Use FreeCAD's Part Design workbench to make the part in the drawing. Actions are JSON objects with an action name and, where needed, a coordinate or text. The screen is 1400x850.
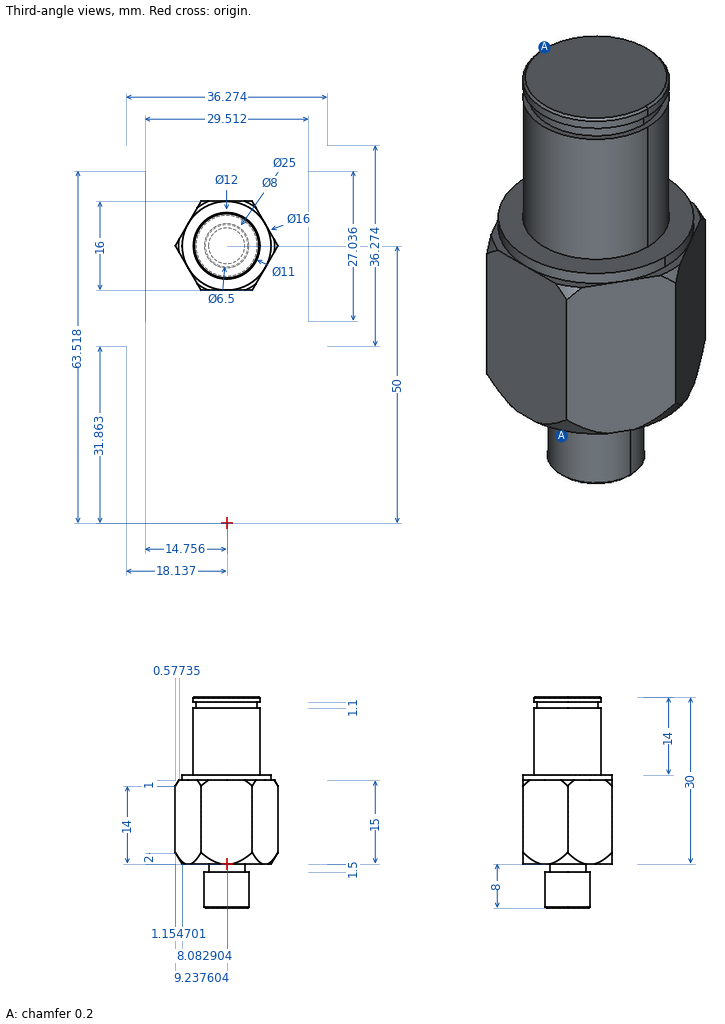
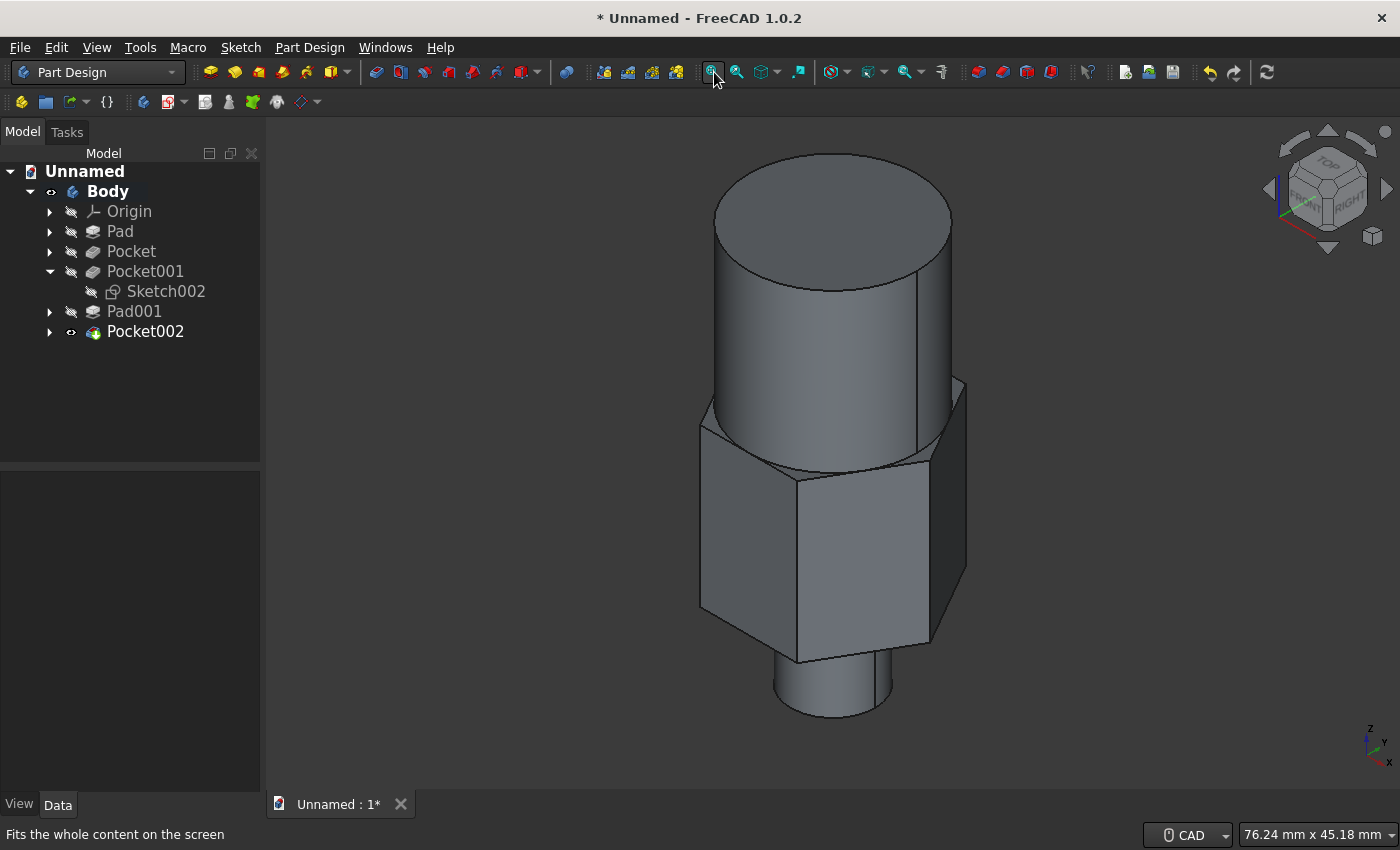
{"action": "left_click", "coordinate": [833, 221]}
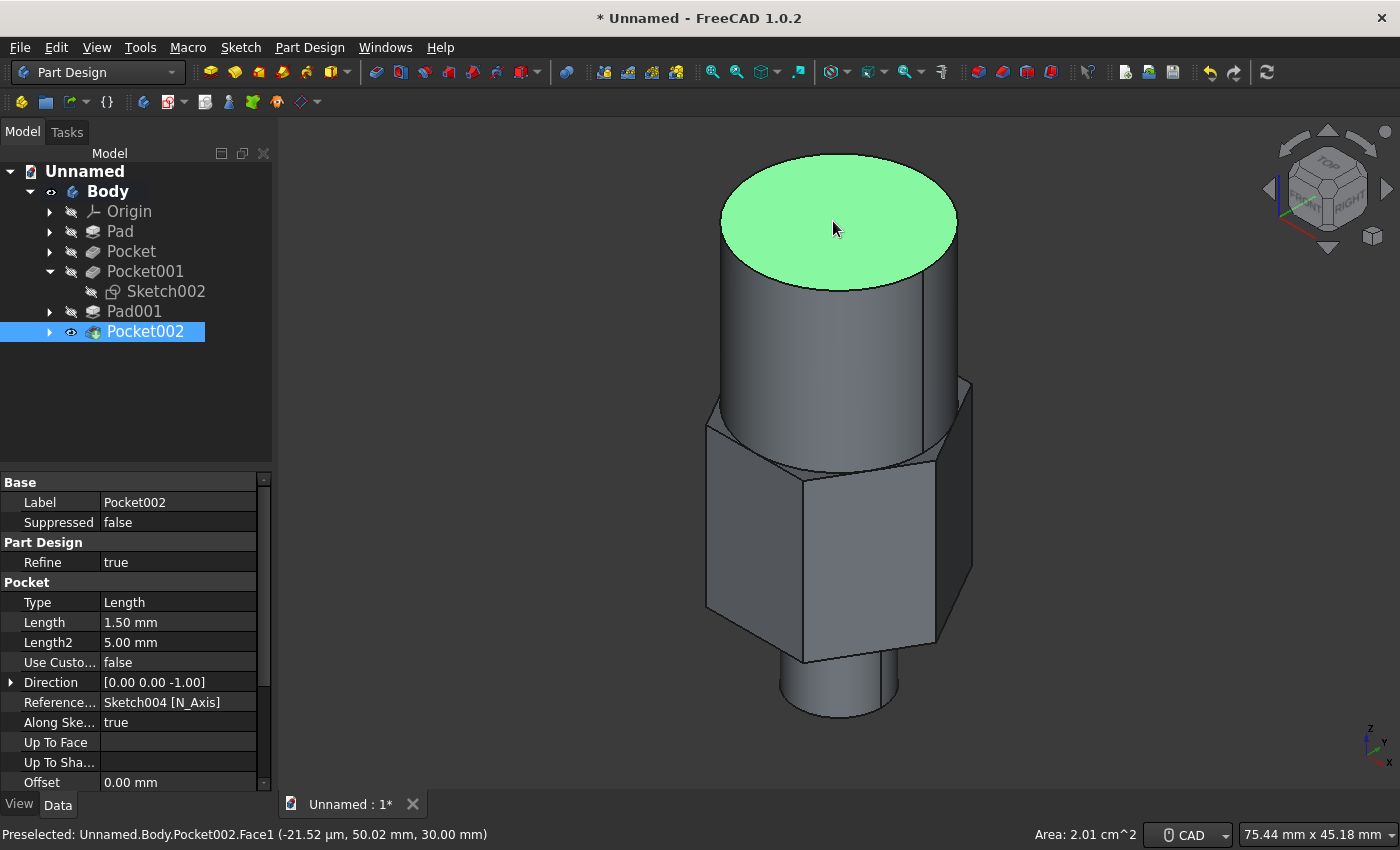
{"action": "left_click", "coordinate": [168, 102]}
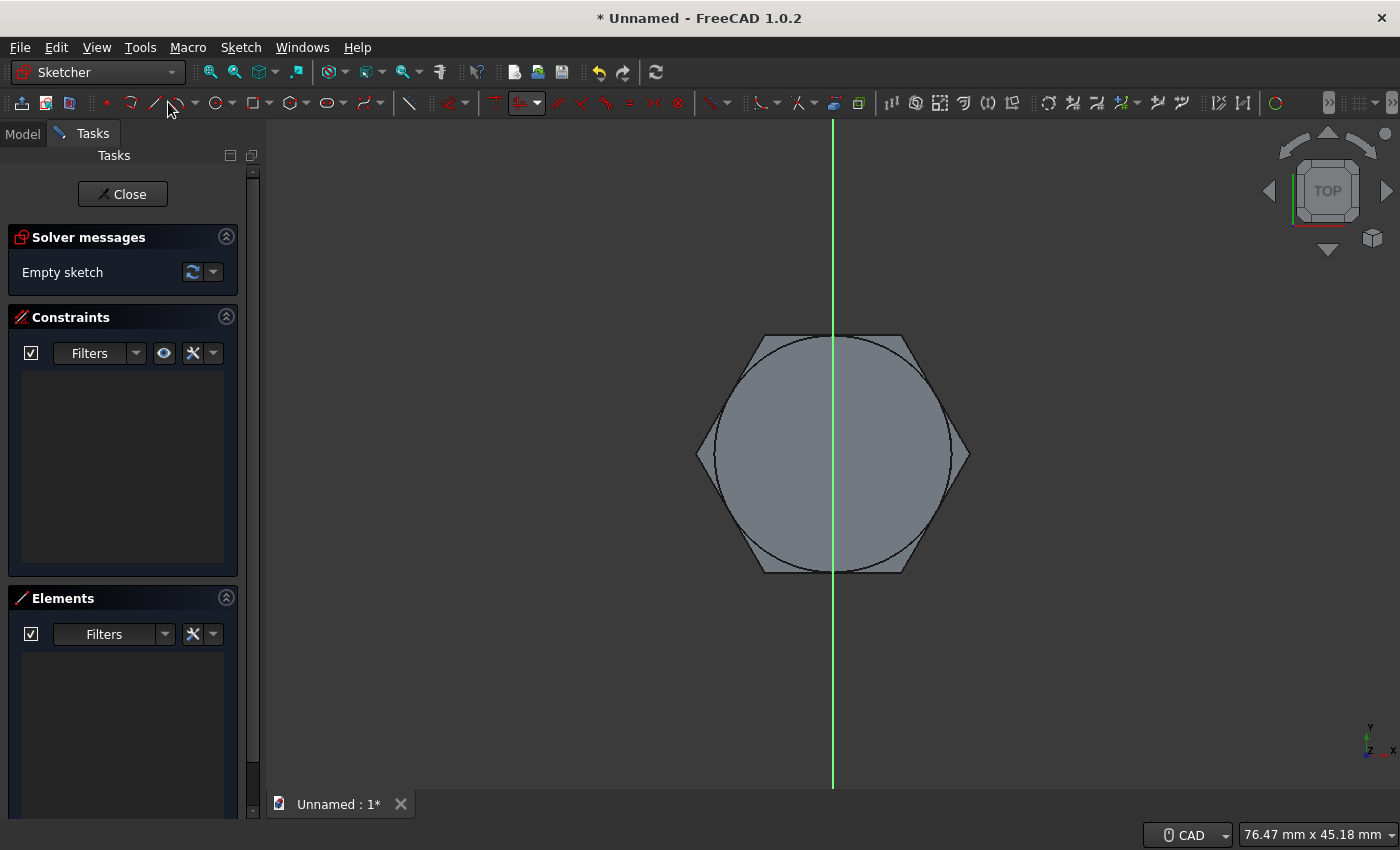
{"action": "scroll", "coordinate": [709, 233], "scroll_direction": "down", "scroll_amount": 4}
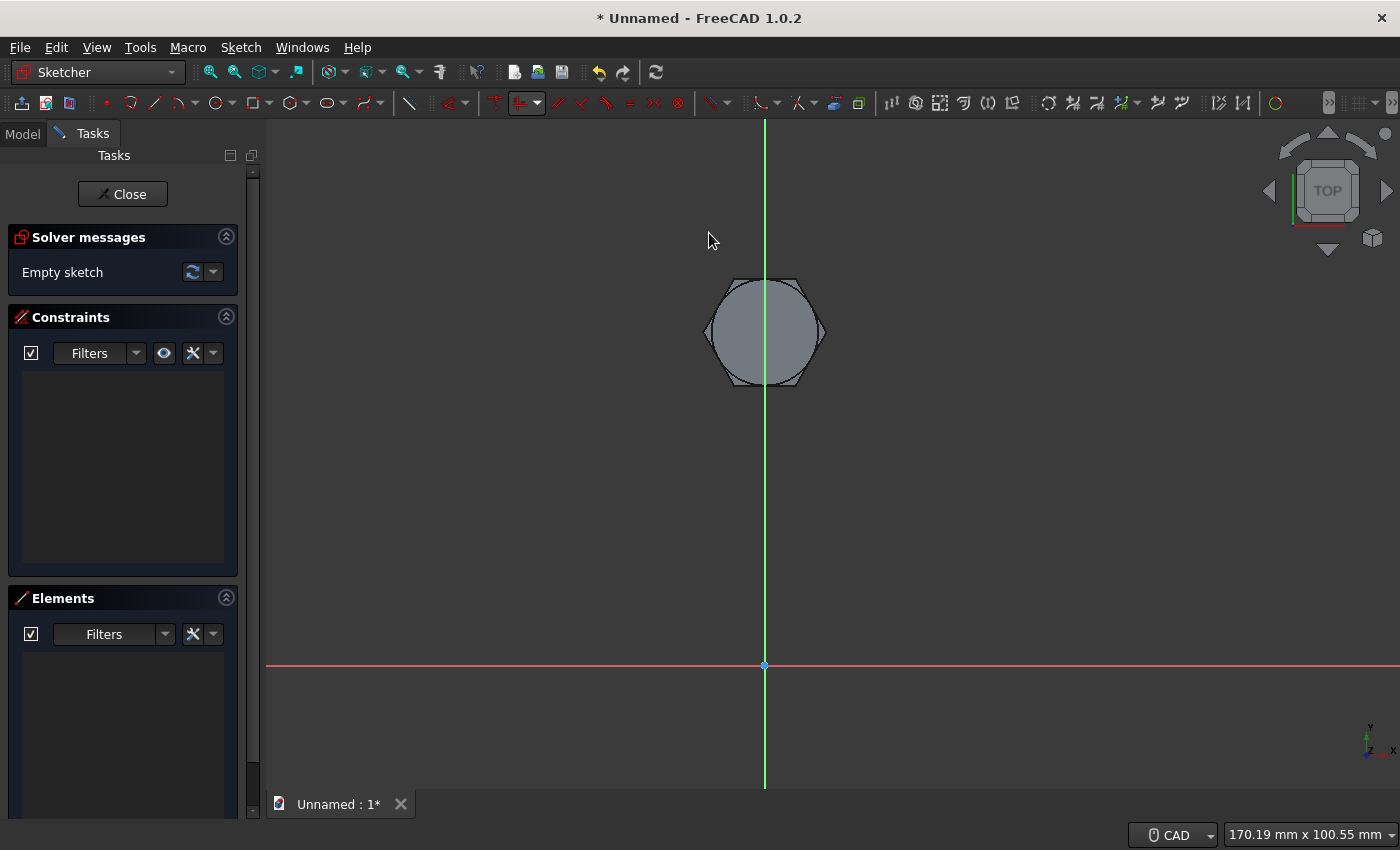
{"action": "left_click", "coordinate": [254, 104]}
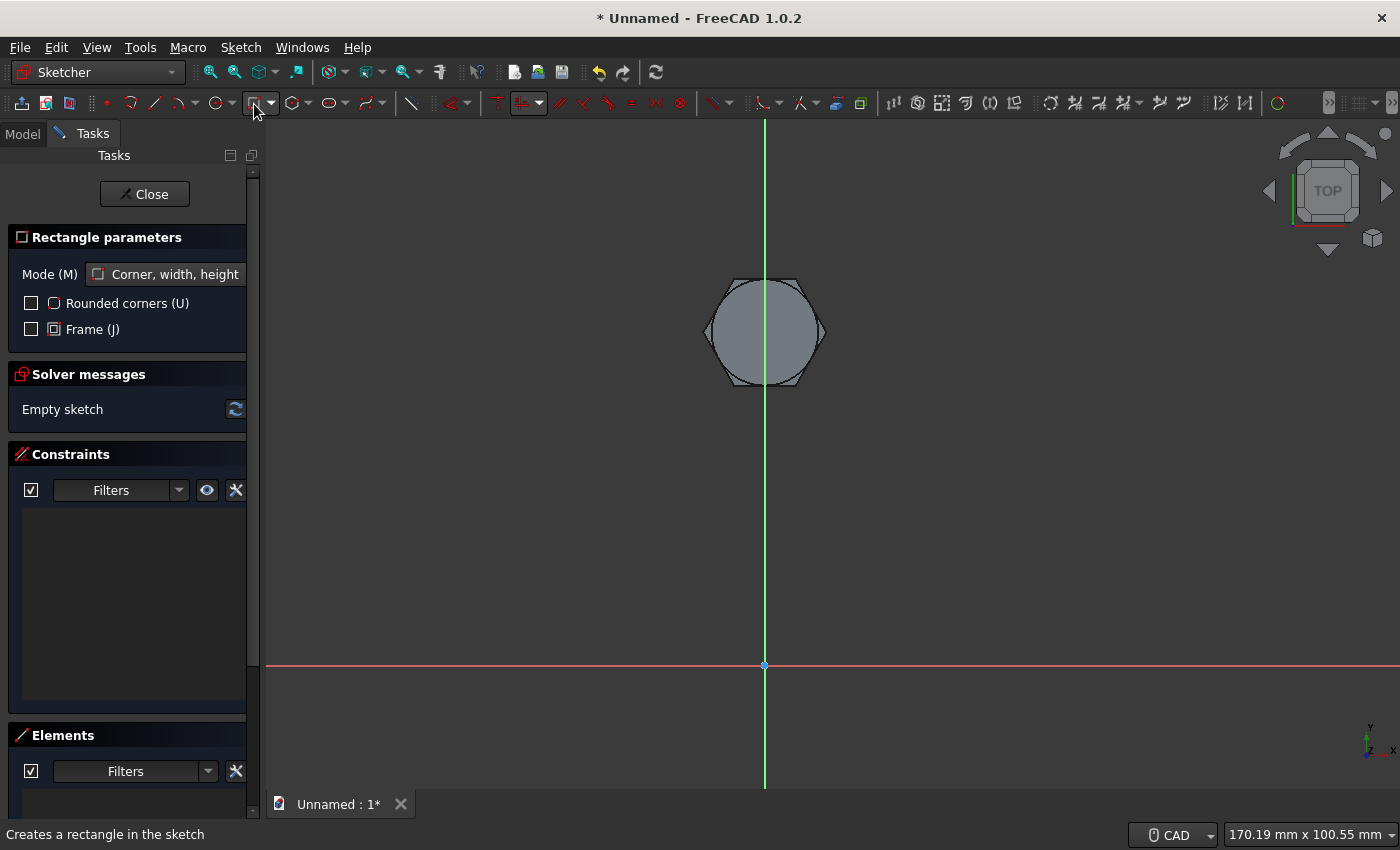
{"action": "left_click", "coordinate": [667, 242]}
{"action": "mouse_move", "coordinate": [863, 422]}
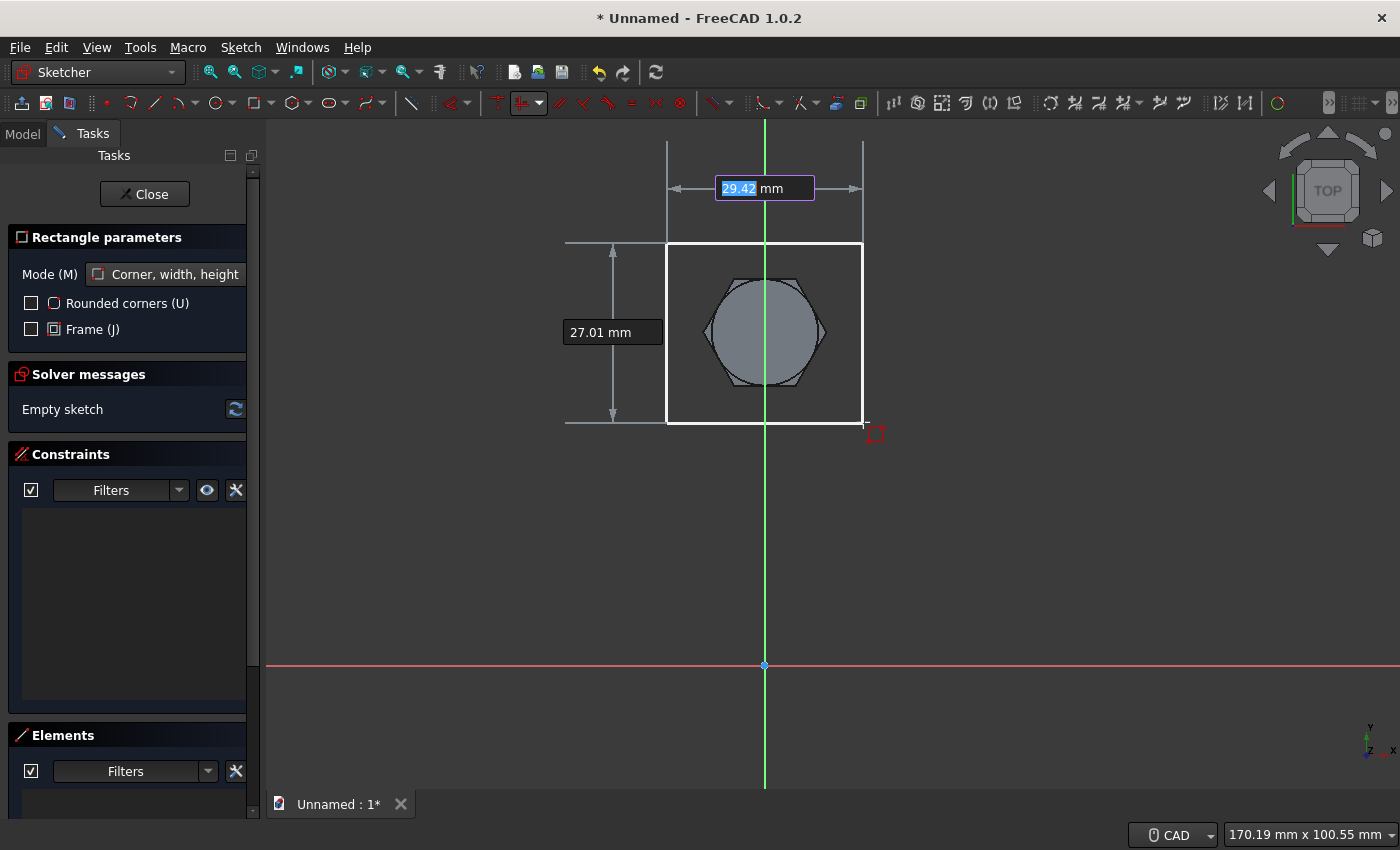
{"action": "type", "text": "29.512"}
{"action": "key", "text": "Tab"}
{"action": "type", "text": "27.036"}
{"action": "key", "text": "Return"}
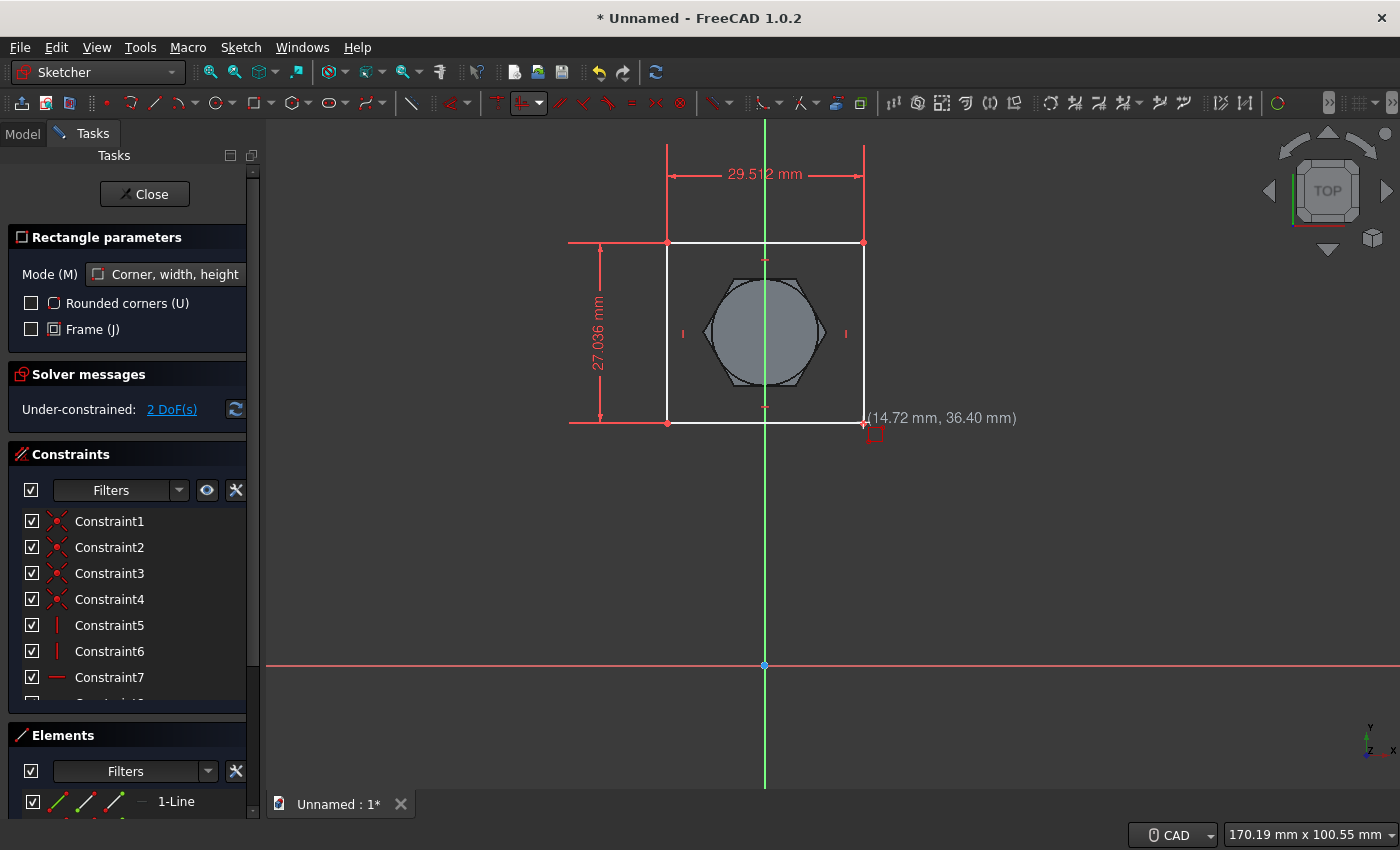
{"action": "left_click", "coordinate": [216, 104]}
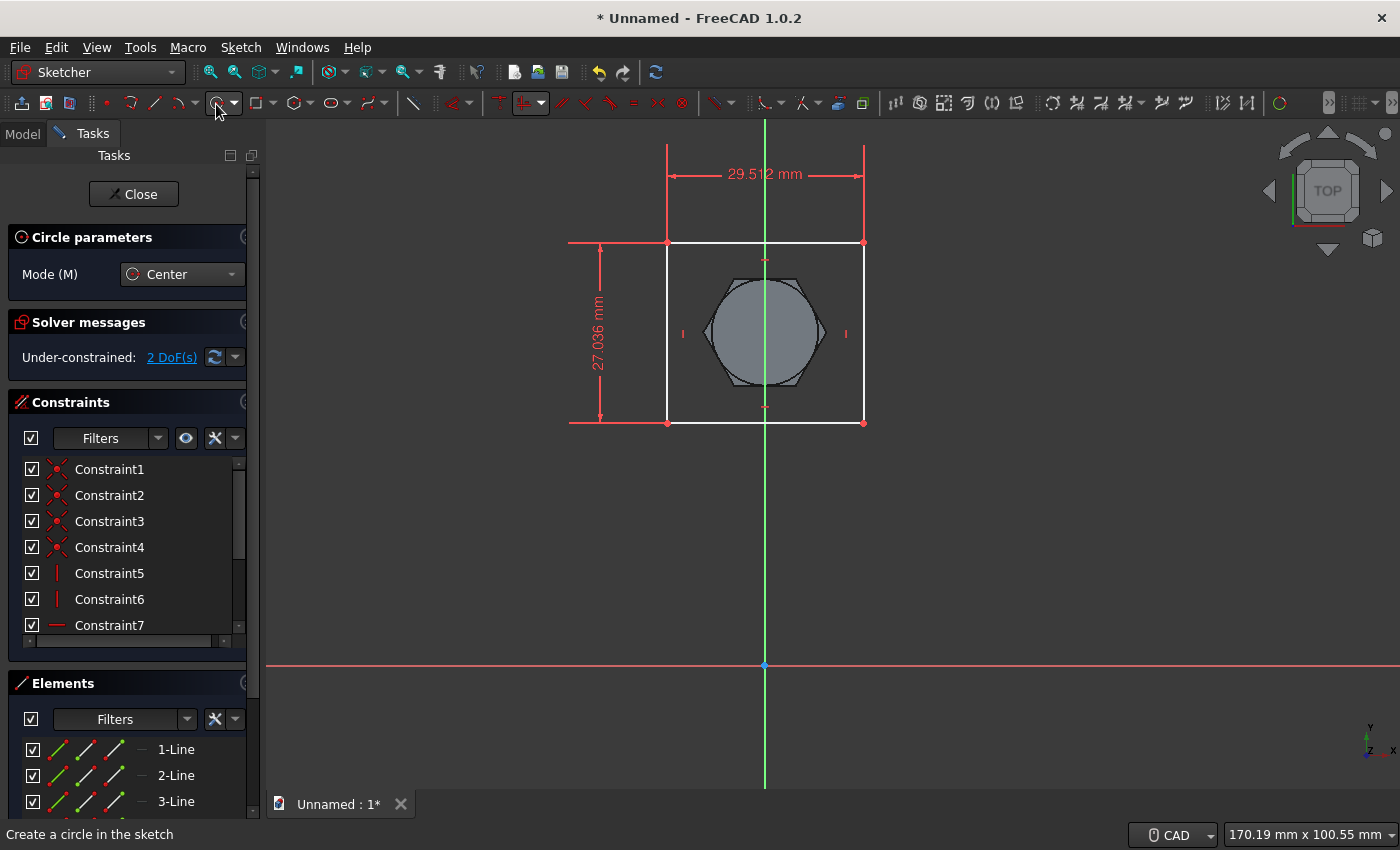
{"action": "left_click", "coordinate": [765, 332]}
{"action": "mouse_move", "coordinate": [793, 304]}